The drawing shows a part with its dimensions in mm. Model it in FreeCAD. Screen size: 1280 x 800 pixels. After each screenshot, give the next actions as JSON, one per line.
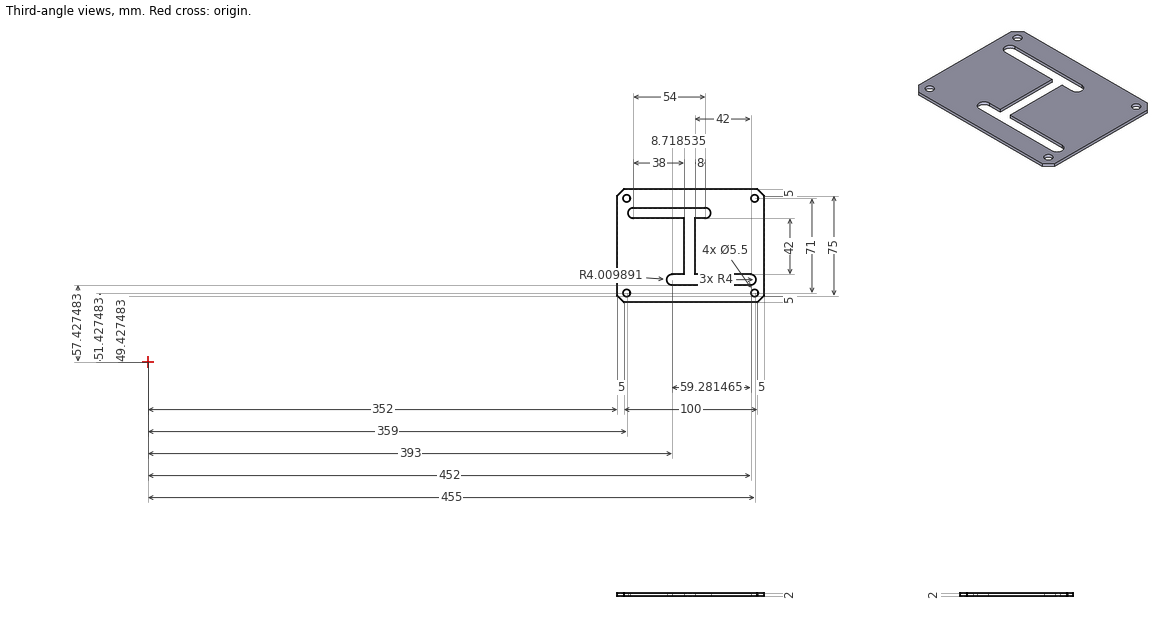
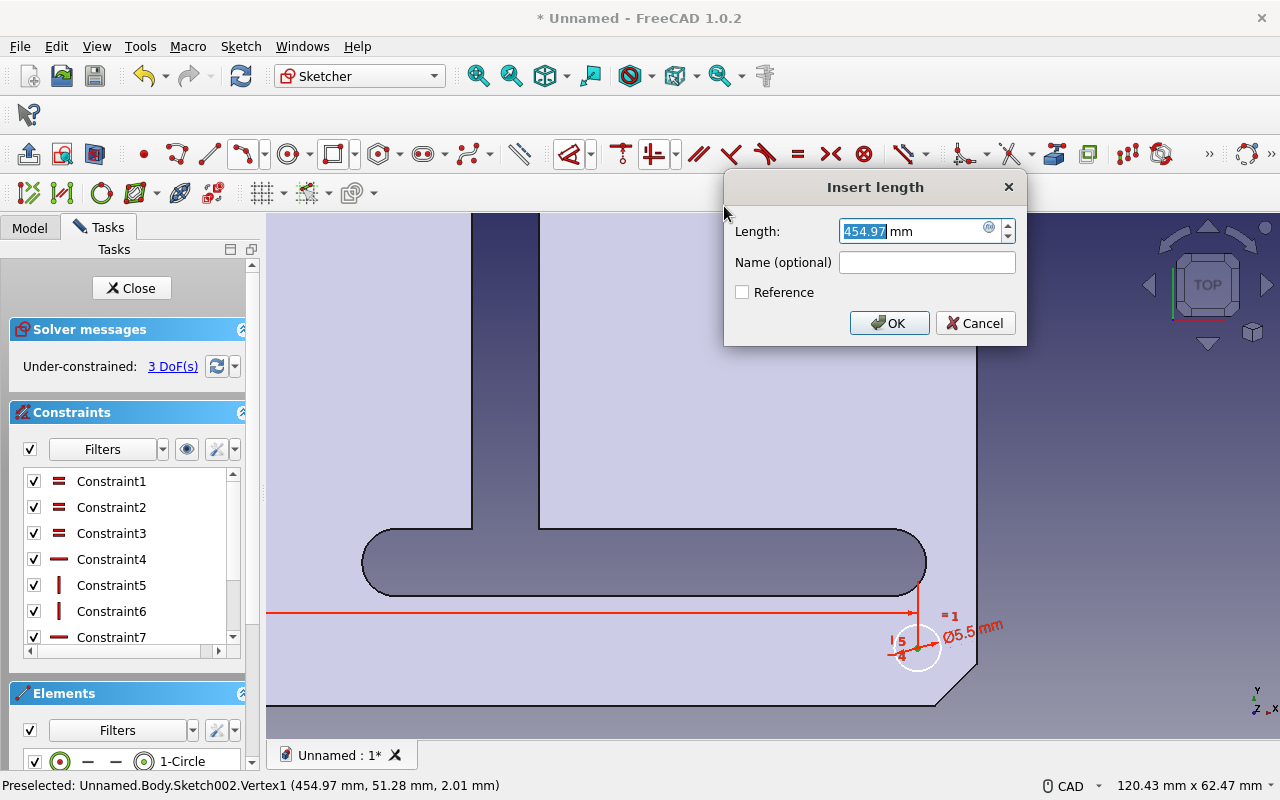
{"action": "type", "text": "455"}
{"action": "key", "text": "Return"}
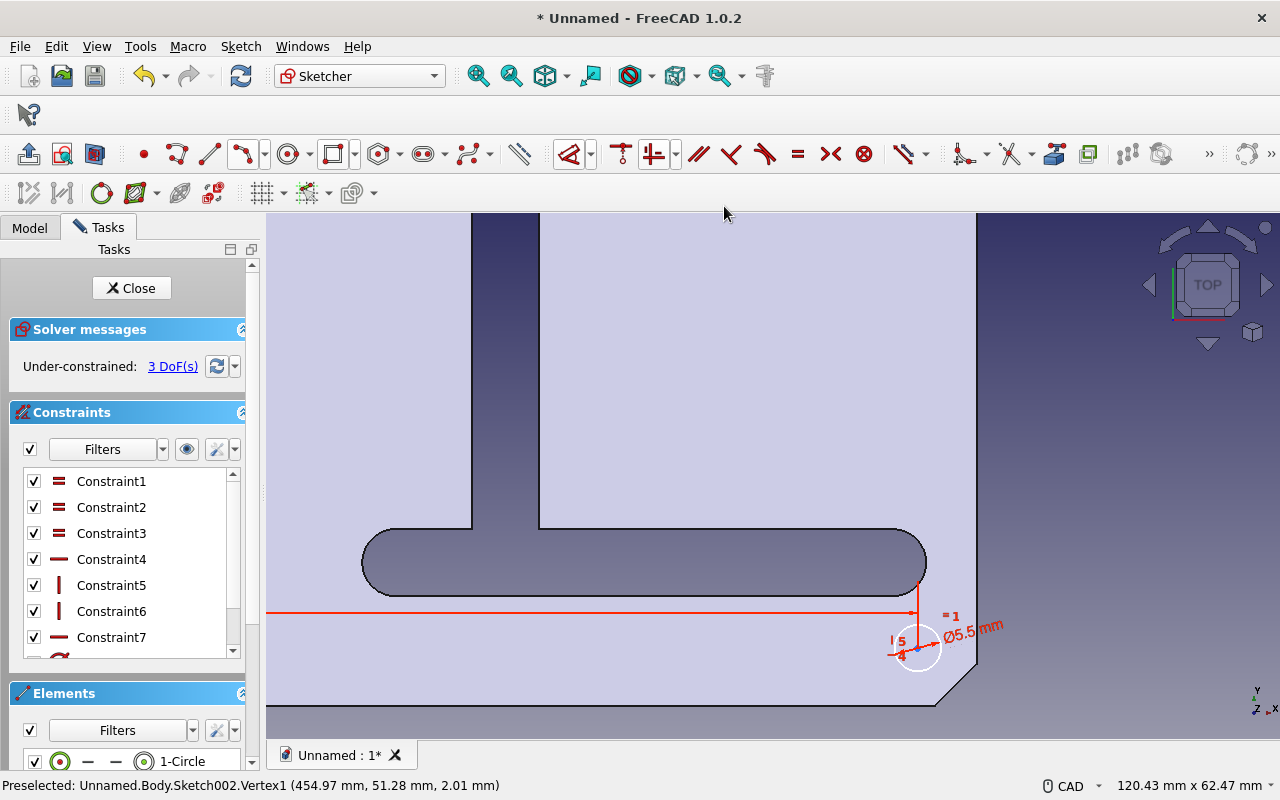
{"action": "scroll", "coordinate": [937, 632], "scroll_direction": "down", "scroll_amount": 3}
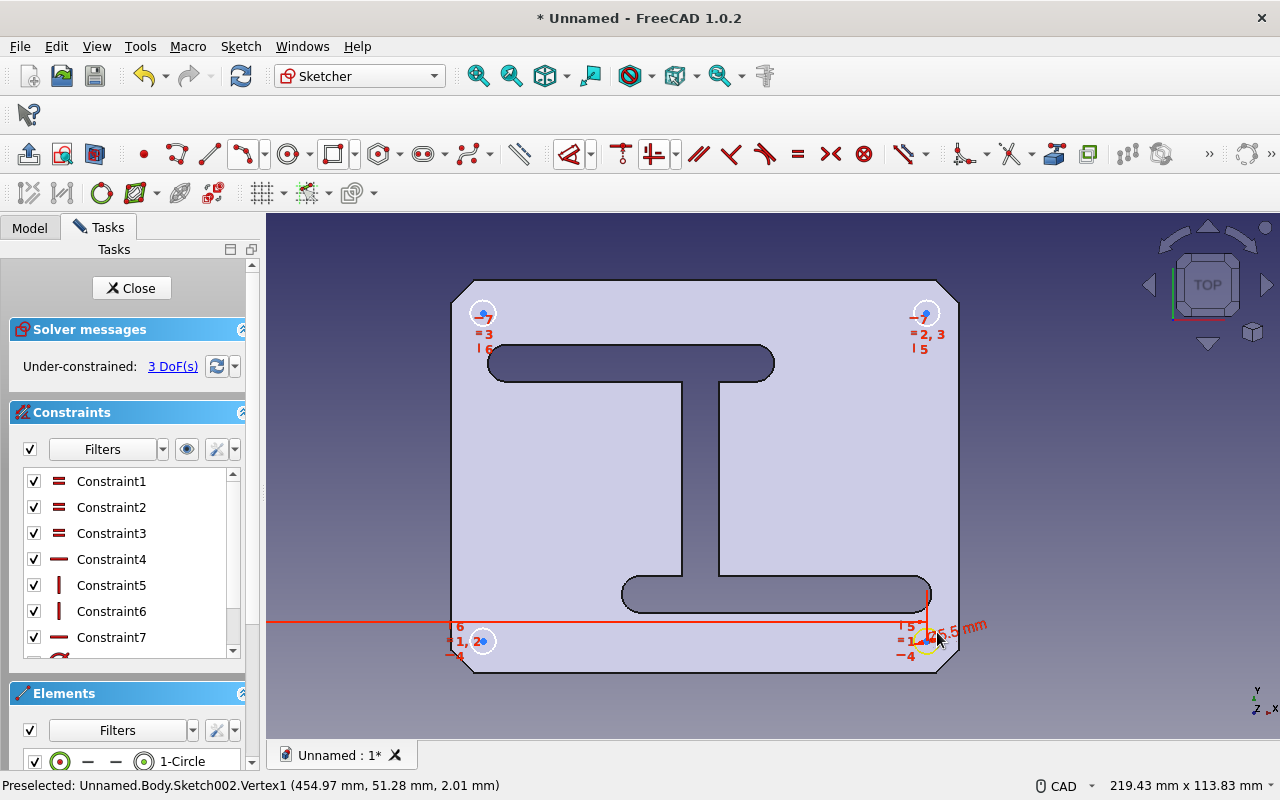
{"action": "left_click", "coordinate": [483, 641]}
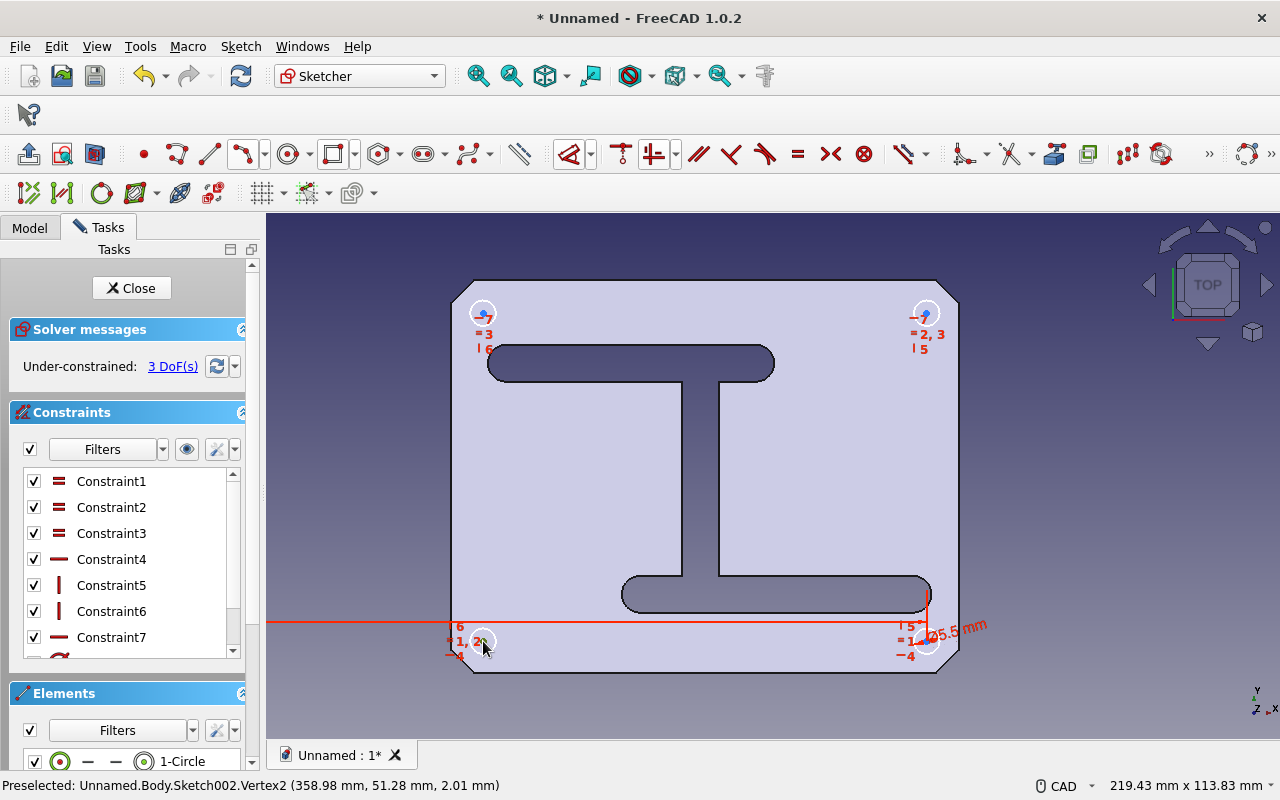
{"action": "left_click", "coordinate": [590, 154]}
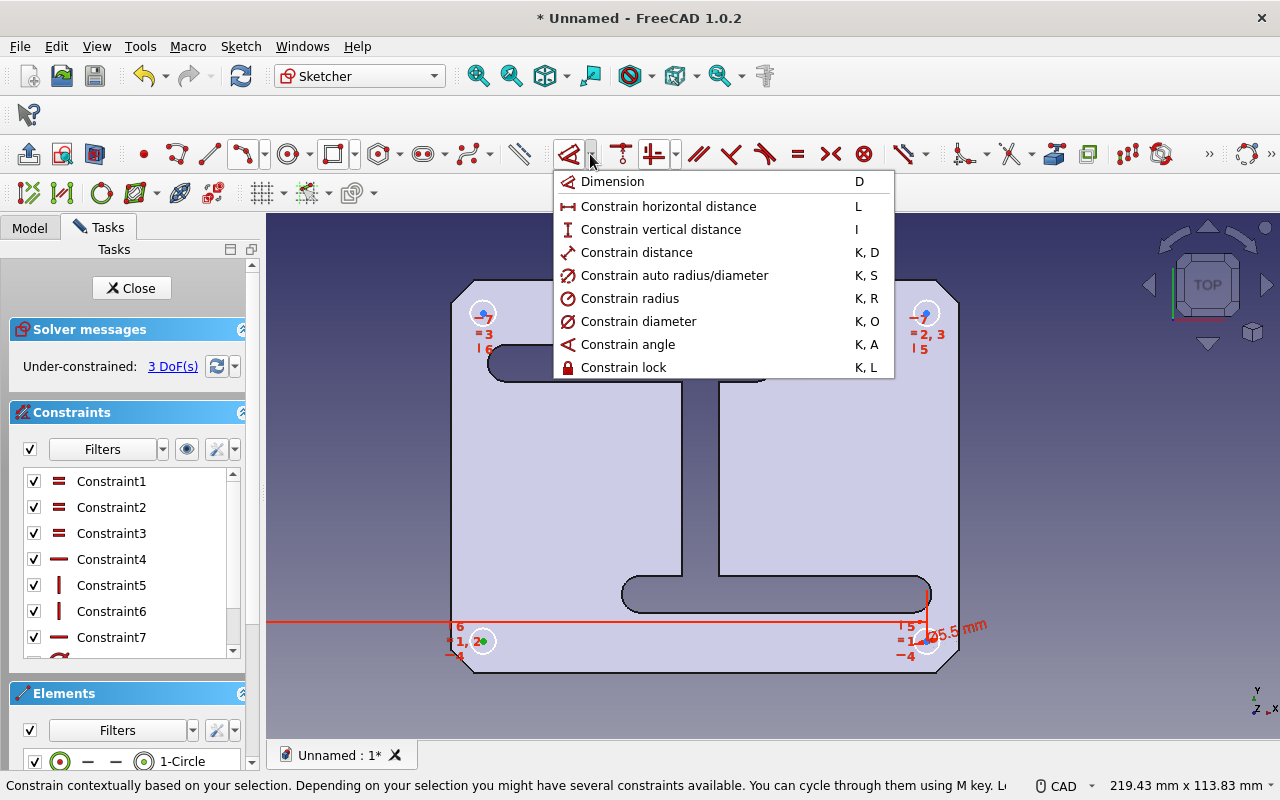
{"action": "left_click", "coordinate": [724, 206]}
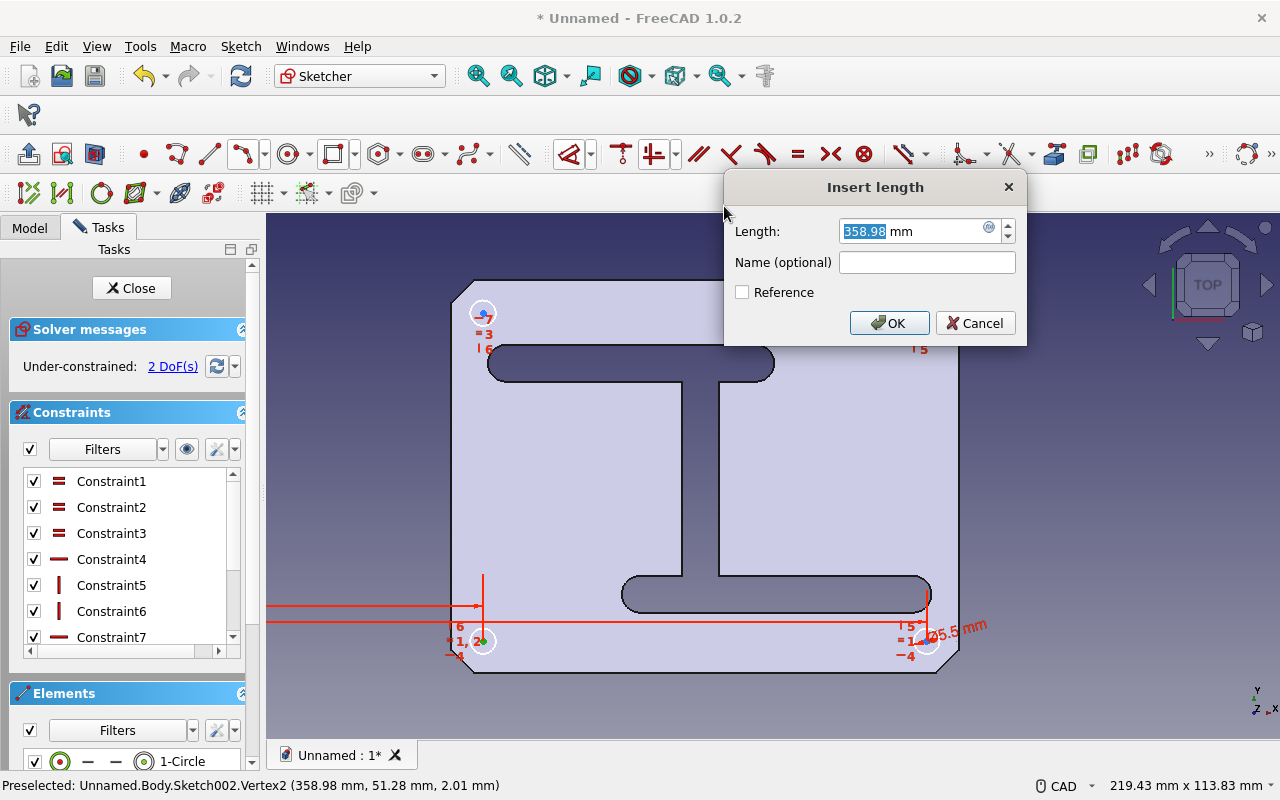
{"action": "type", "text": "359"}
{"action": "key", "text": "Return"}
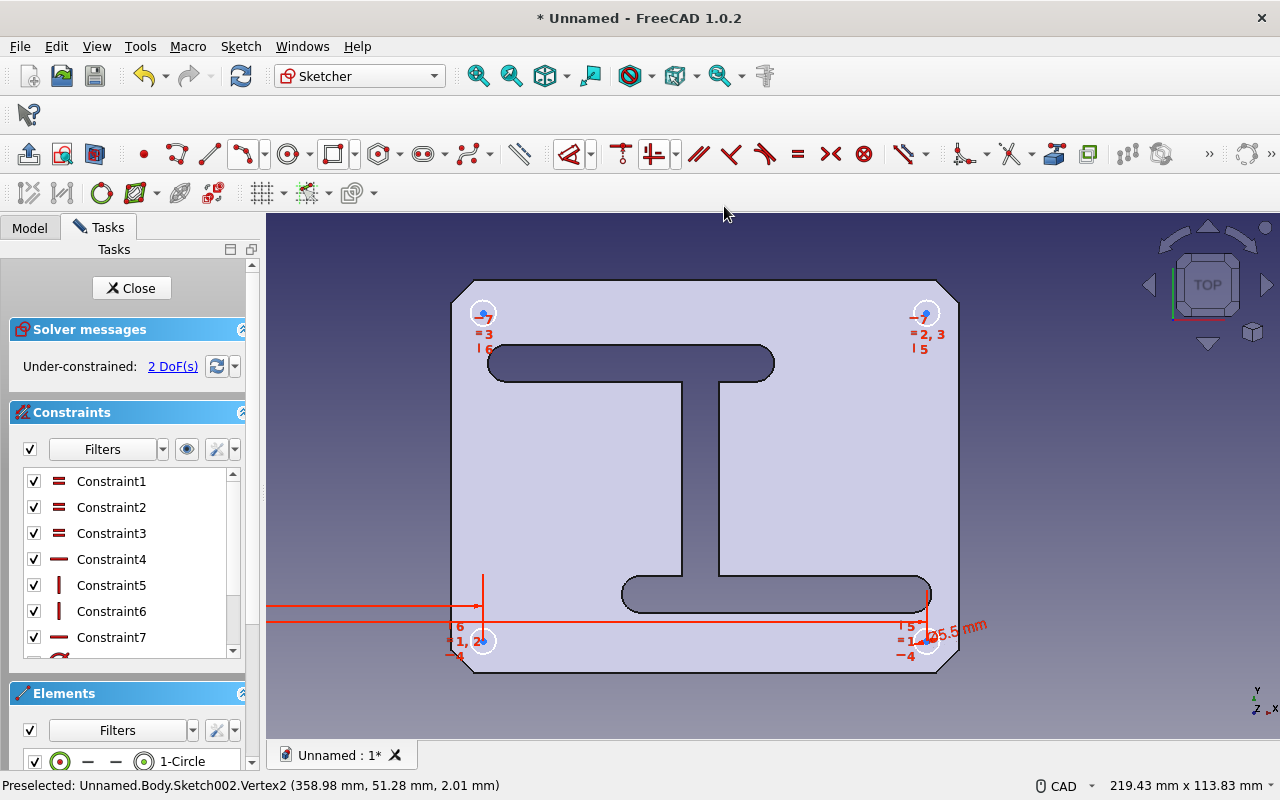
{"action": "left_click", "coordinate": [927, 641]}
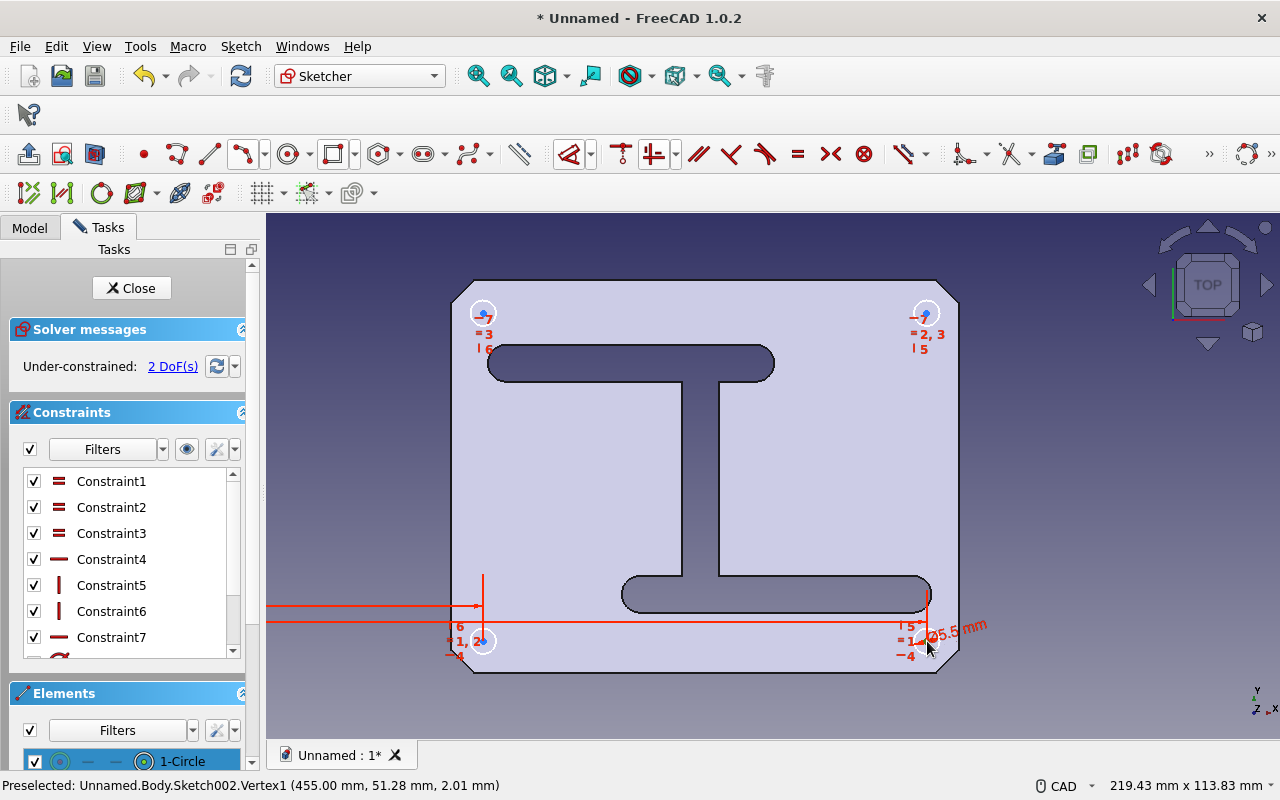
{"action": "left_click", "coordinate": [927, 313]}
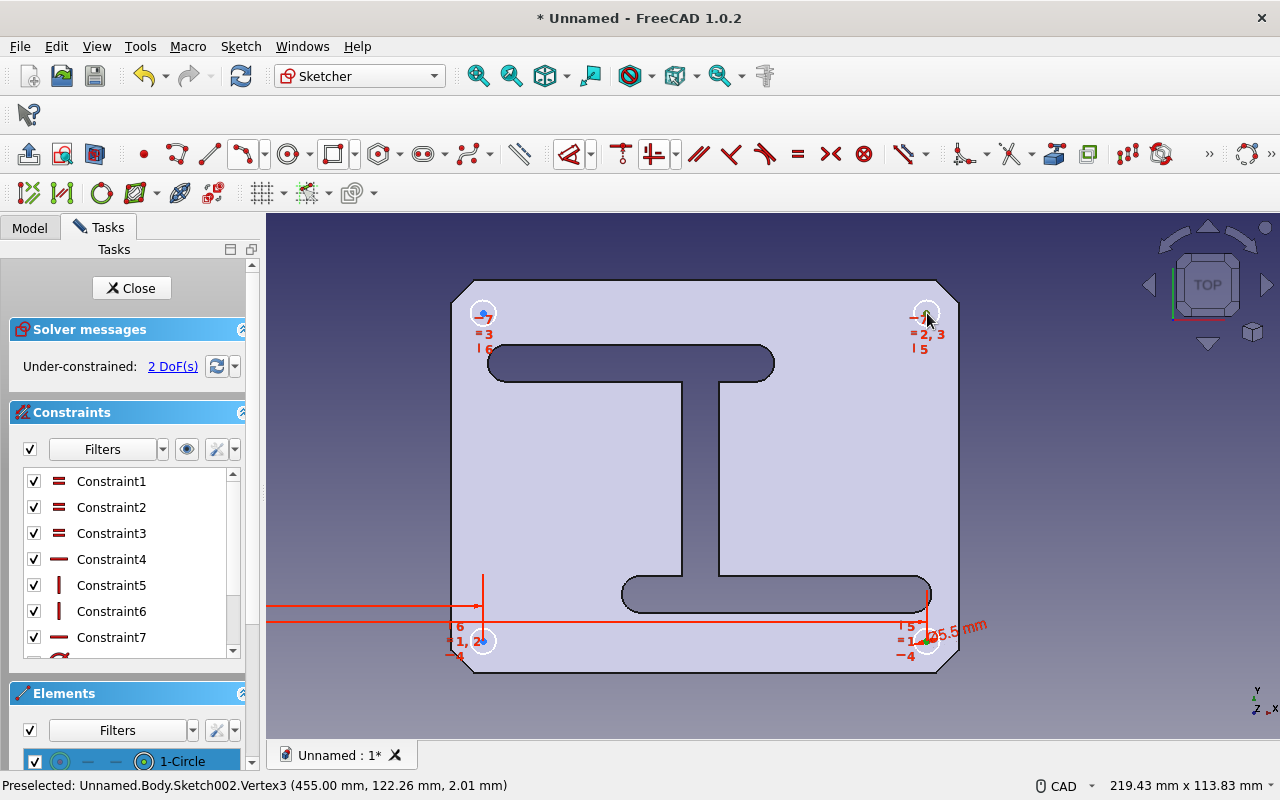
{"action": "key", "text": "i"}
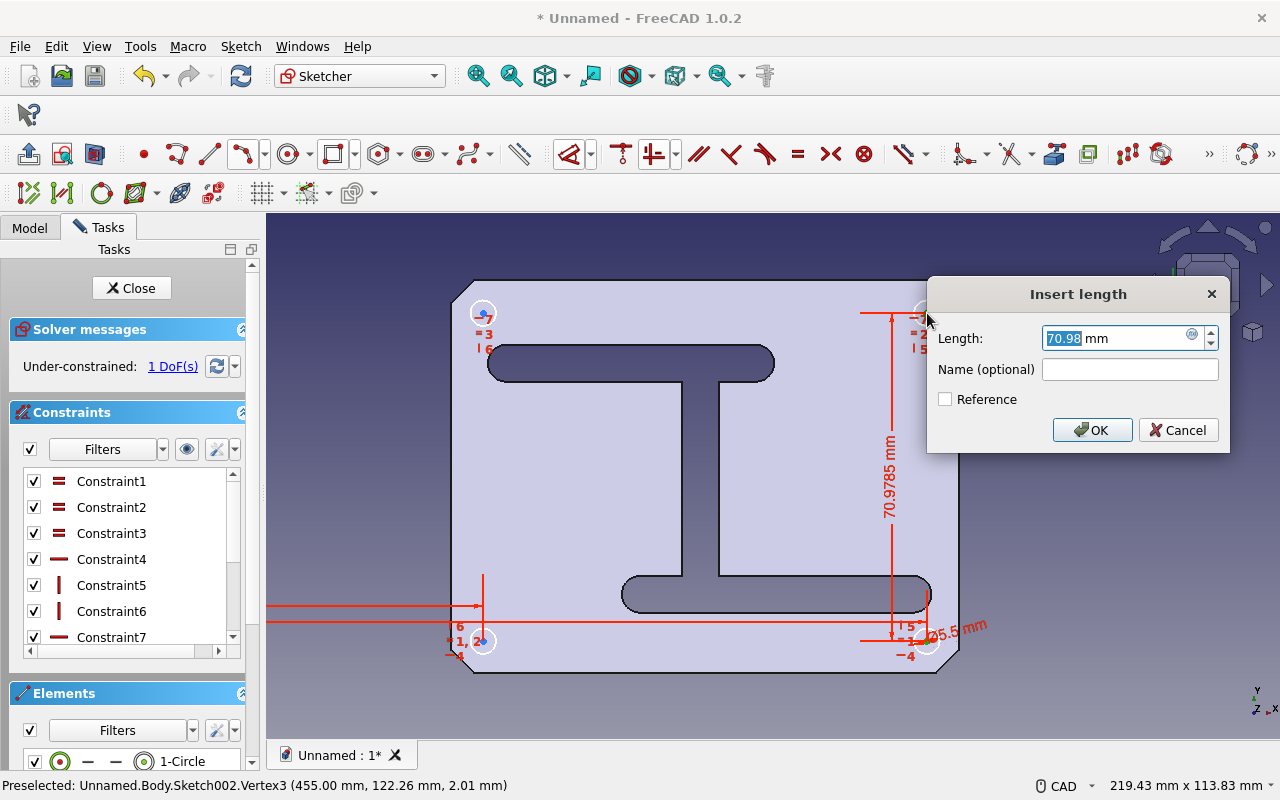
{"action": "type", "text": "71"}
{"action": "key", "text": "Return"}